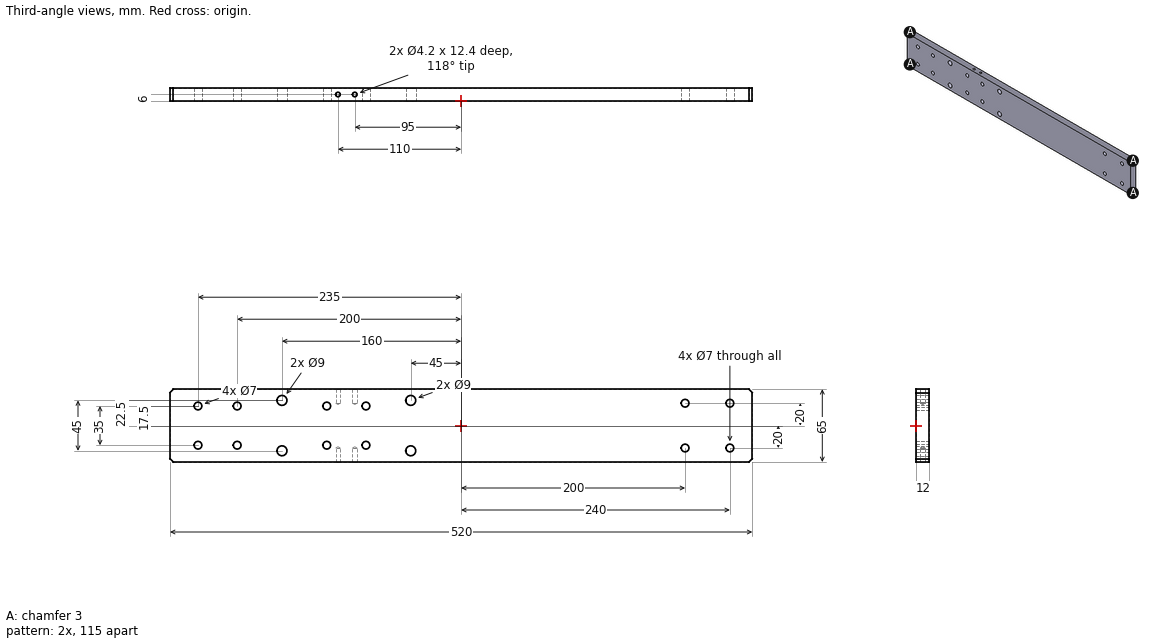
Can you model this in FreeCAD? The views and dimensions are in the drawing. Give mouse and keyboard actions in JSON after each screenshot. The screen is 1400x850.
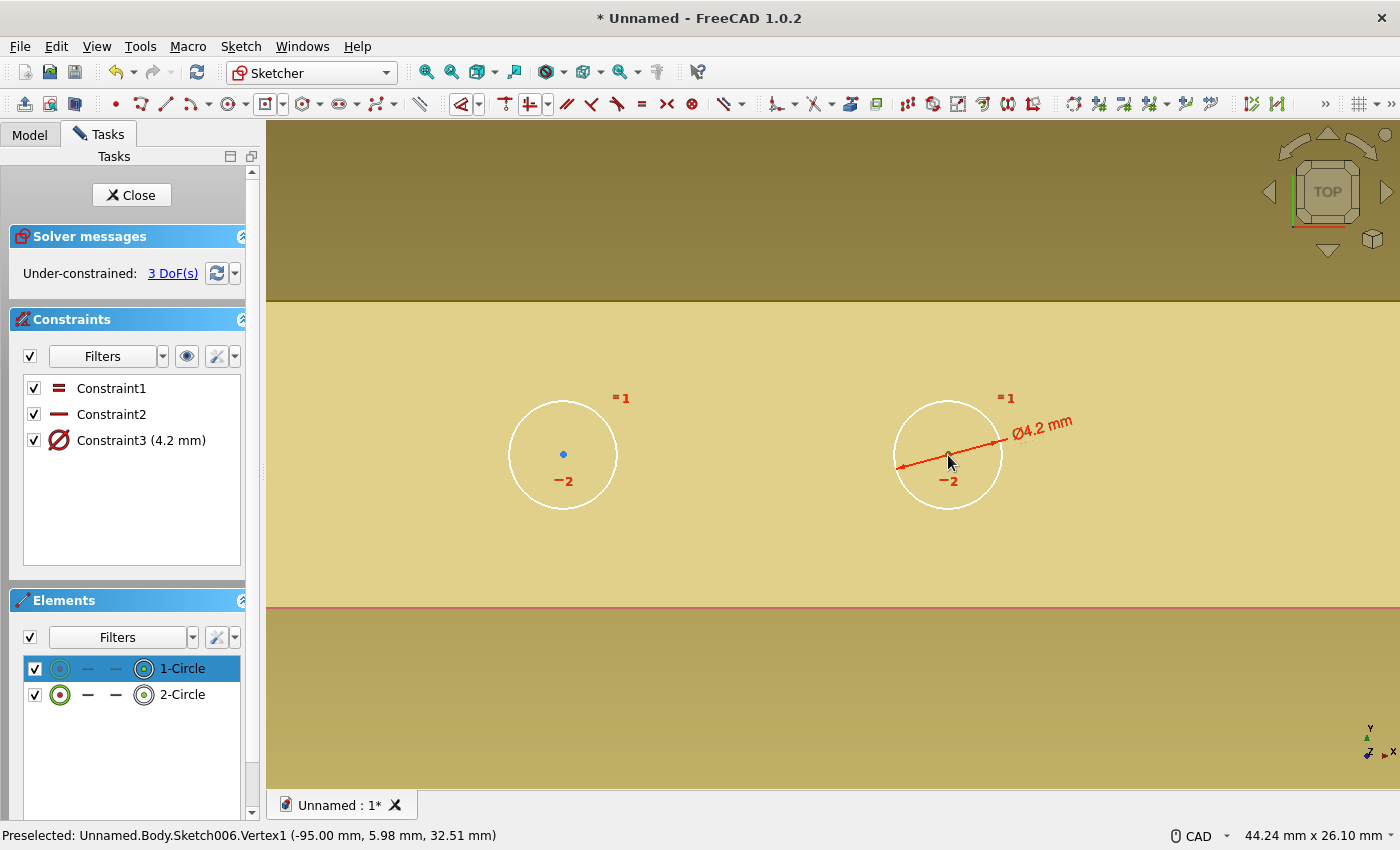
{"action": "left_click", "coordinate": [478, 104]}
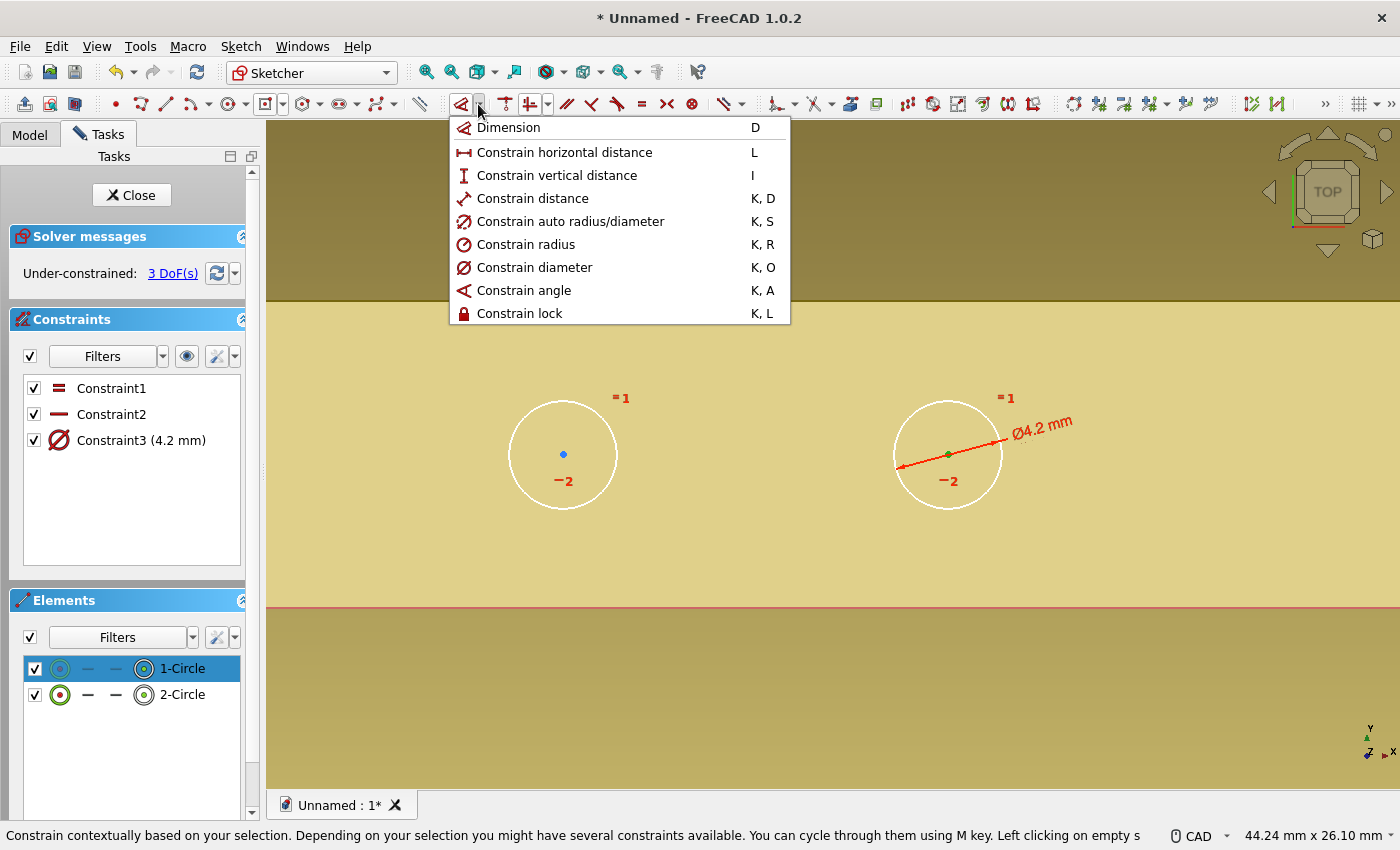
{"action": "left_click", "coordinate": [620, 176]}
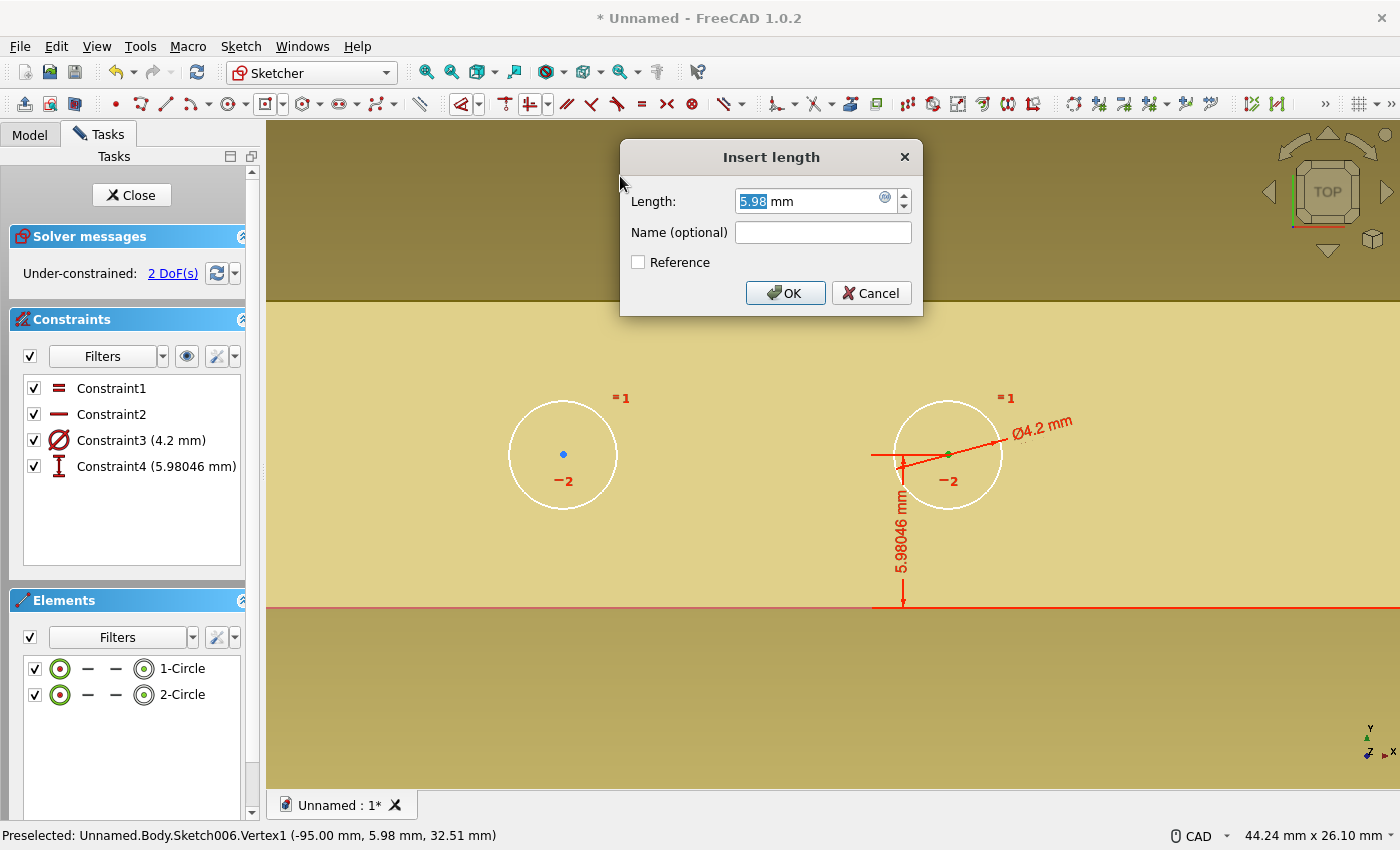
{"action": "type", "text": "6"}
{"action": "key", "text": "Return"}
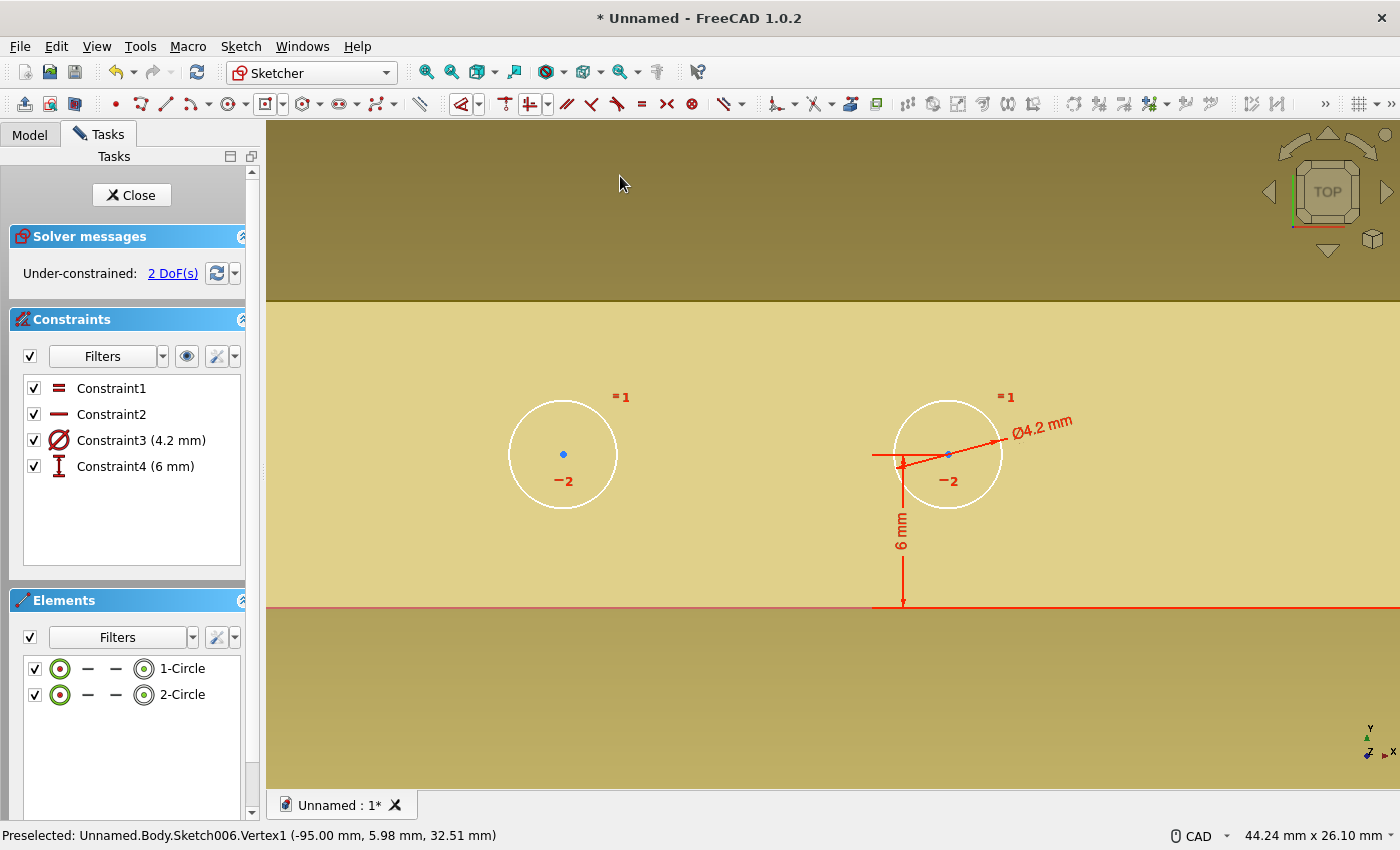
{"action": "left_click", "coordinate": [948, 454]}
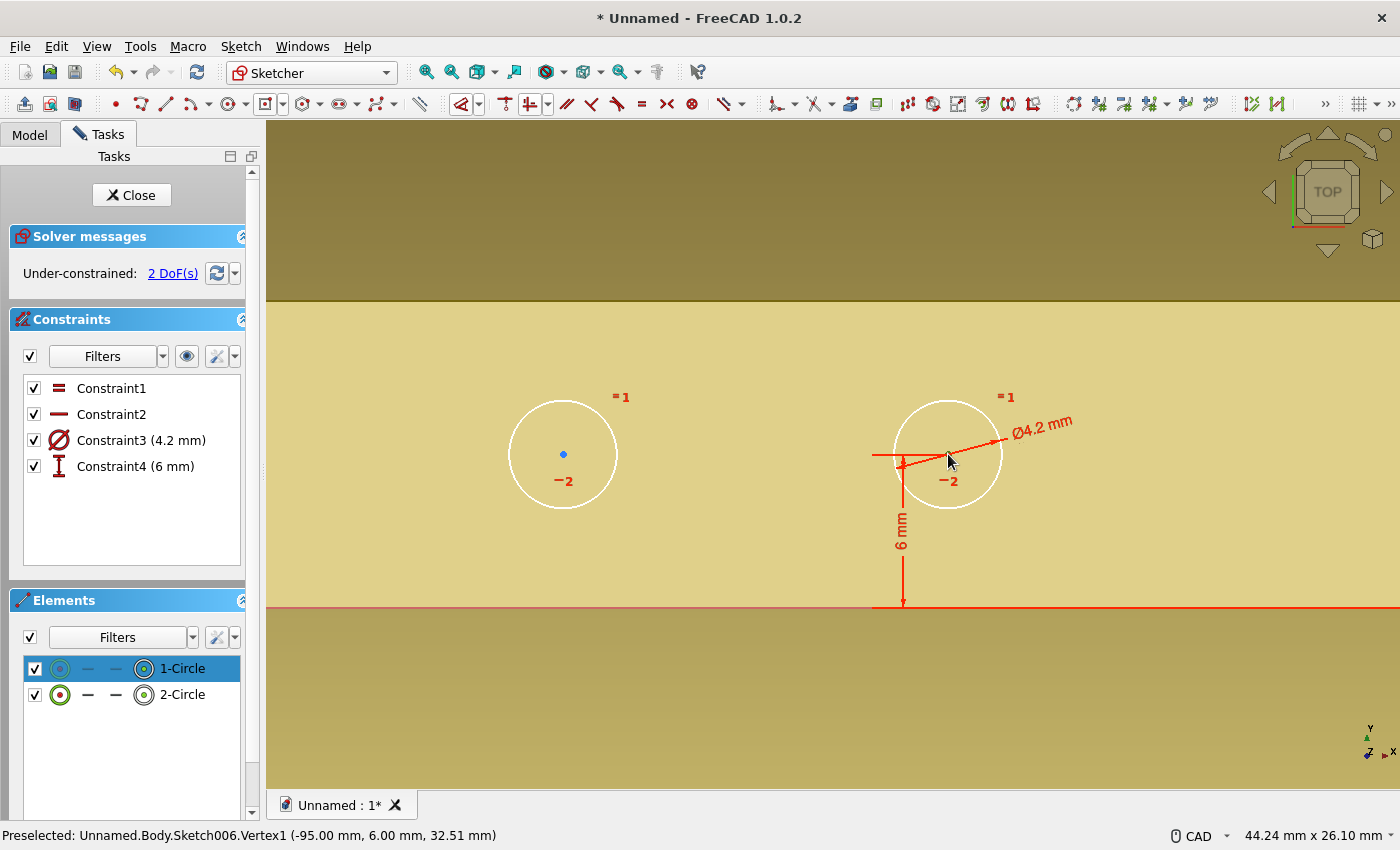
{"action": "key", "text": "l"}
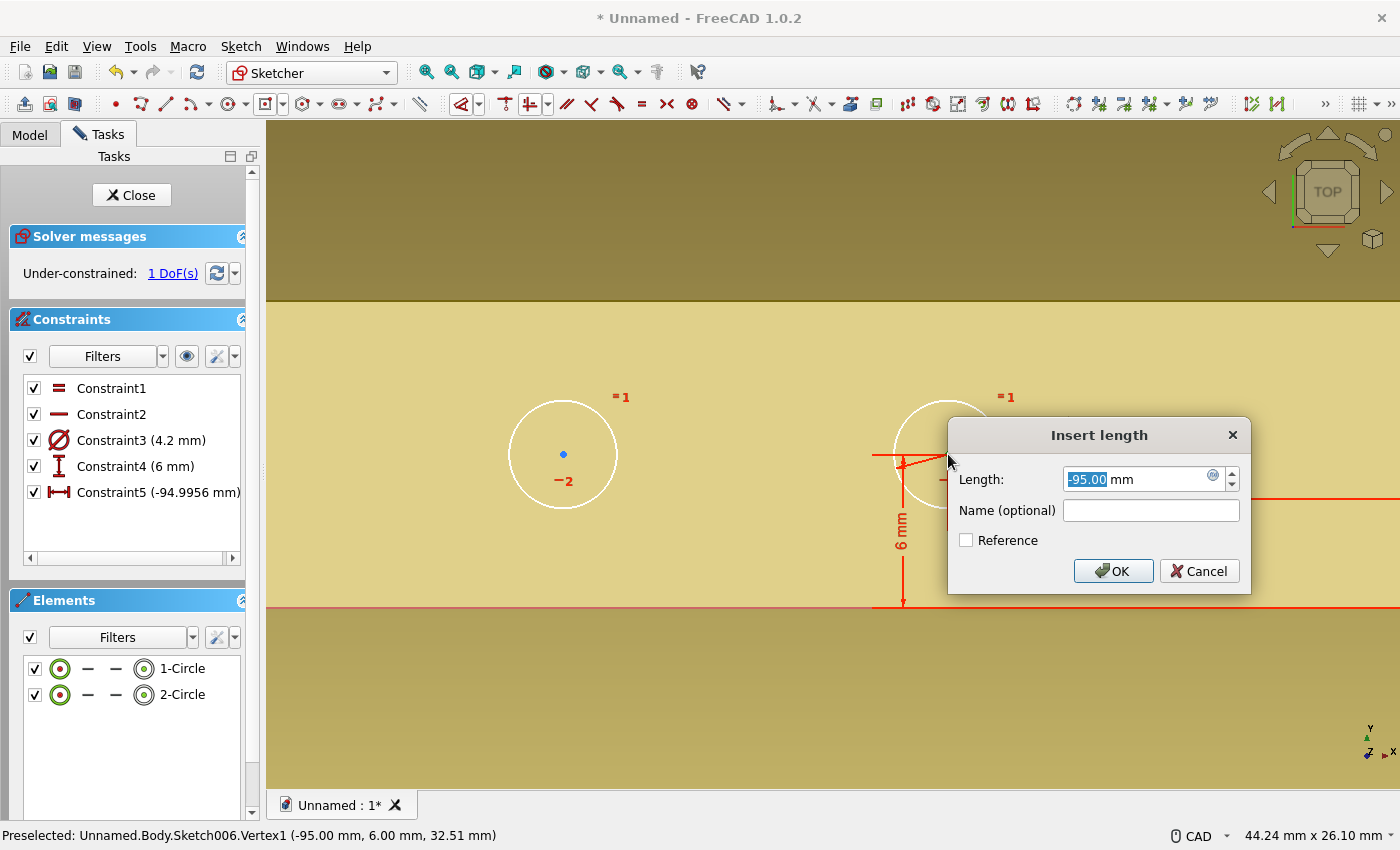
{"action": "type", "text": "-95"}
{"action": "key", "text": "Return"}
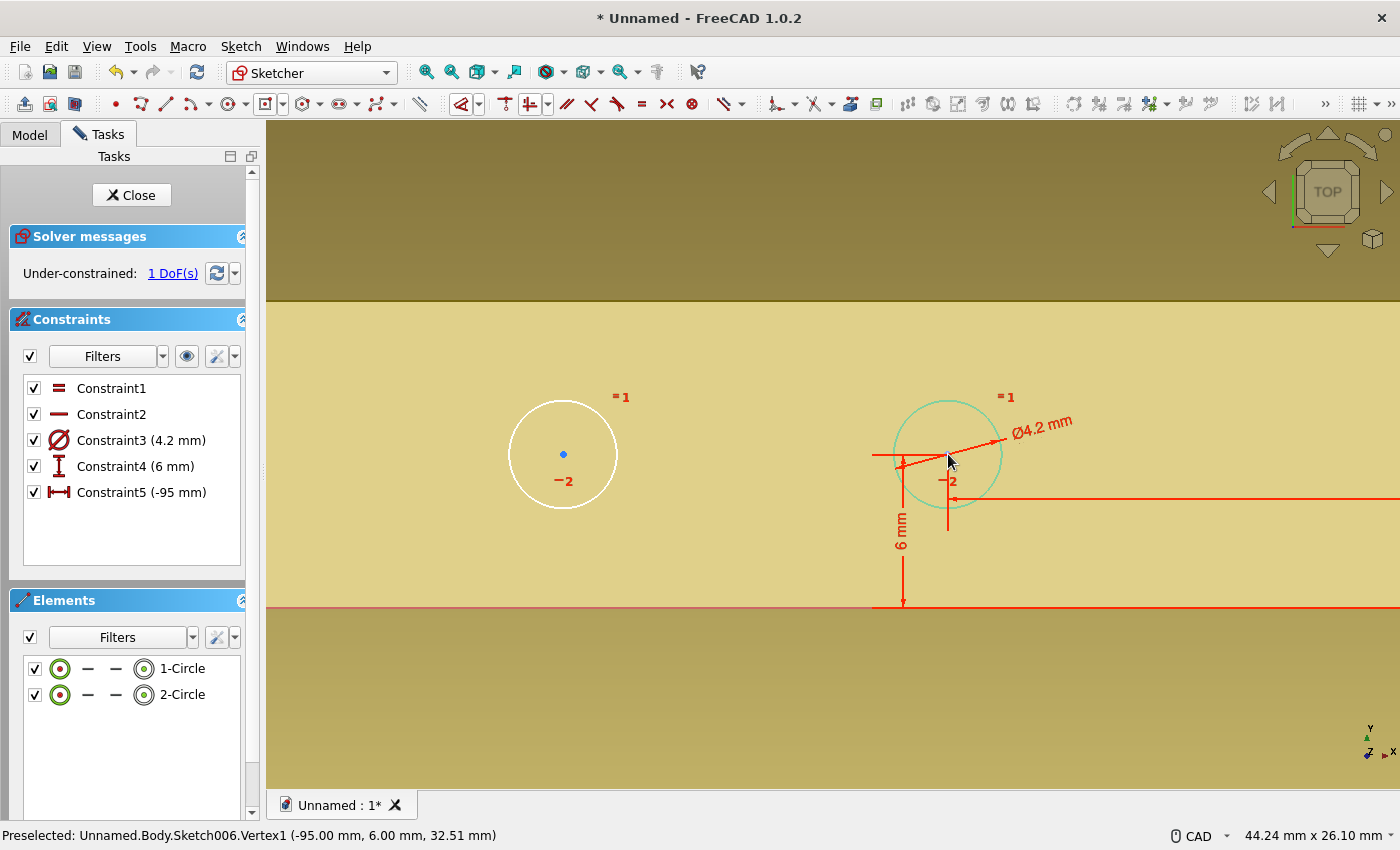
{"action": "left_click", "coordinate": [563, 454]}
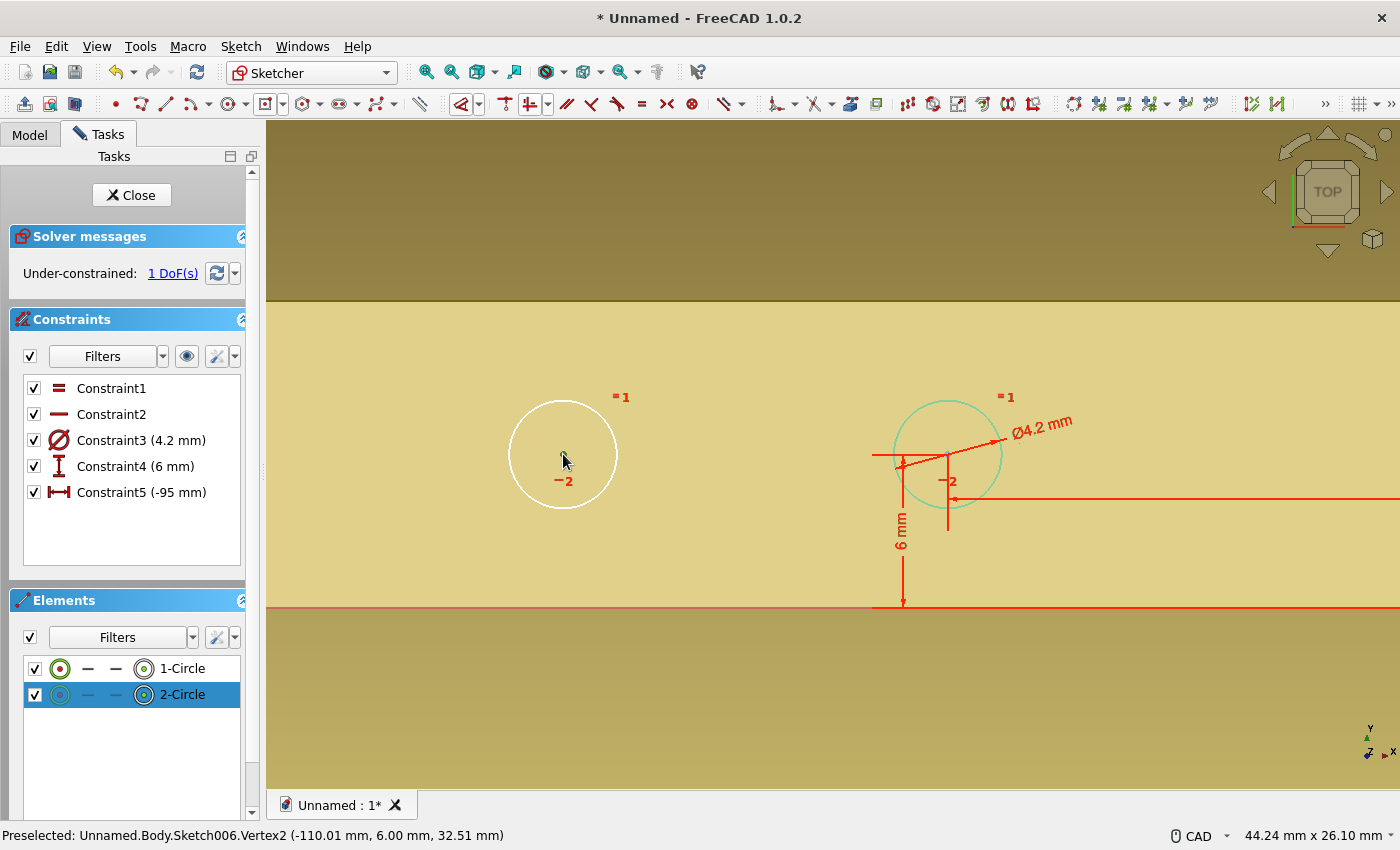
{"action": "left_click", "coordinate": [478, 104]}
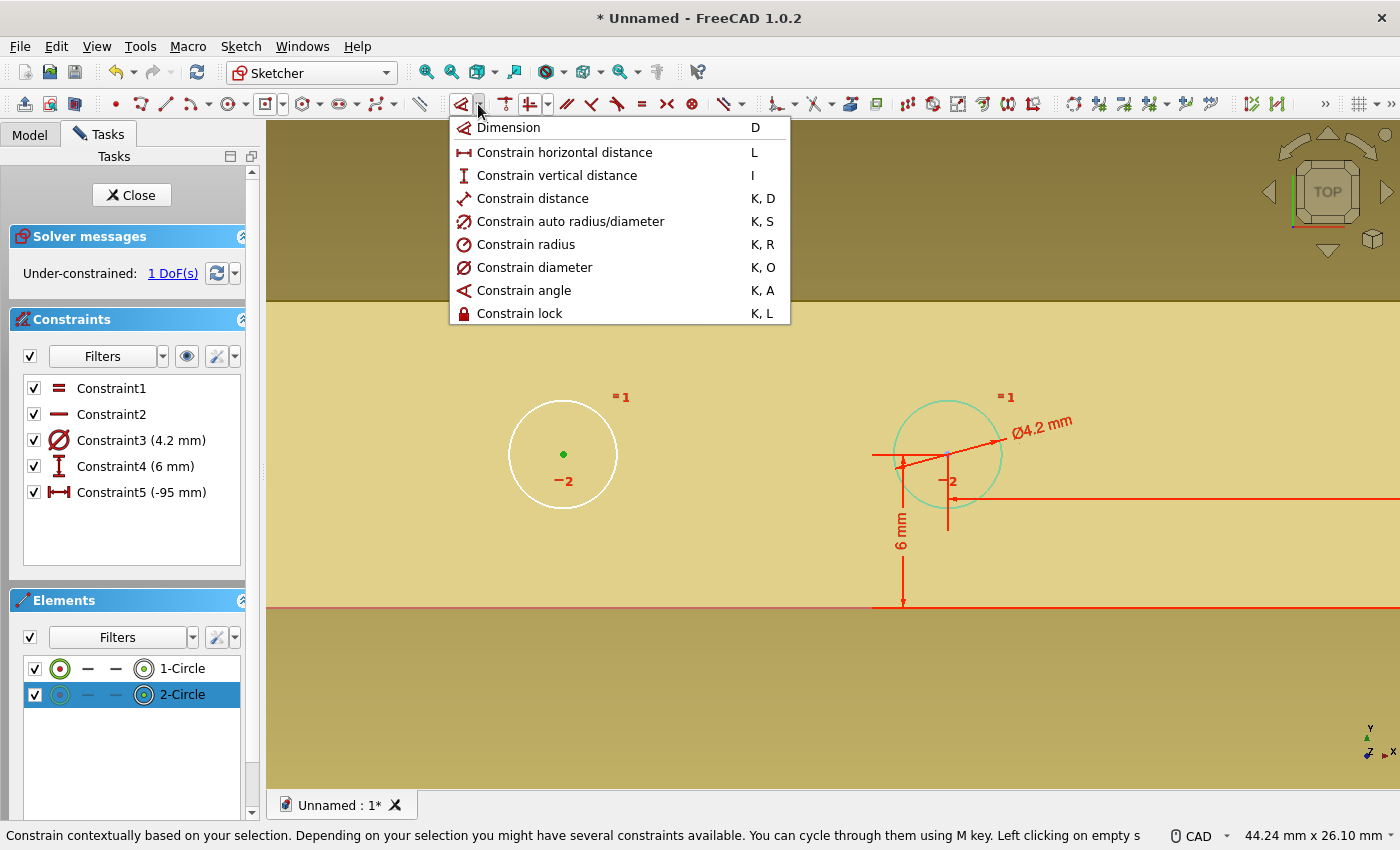
{"action": "left_click", "coordinate": [620, 152]}